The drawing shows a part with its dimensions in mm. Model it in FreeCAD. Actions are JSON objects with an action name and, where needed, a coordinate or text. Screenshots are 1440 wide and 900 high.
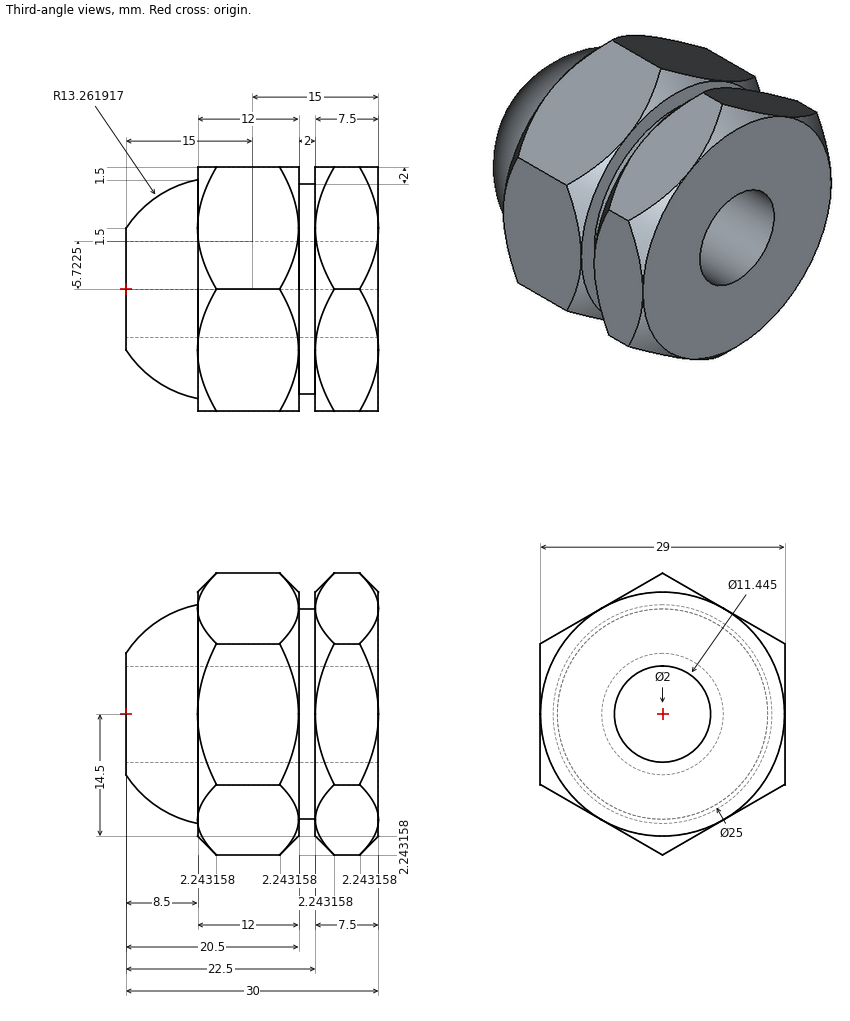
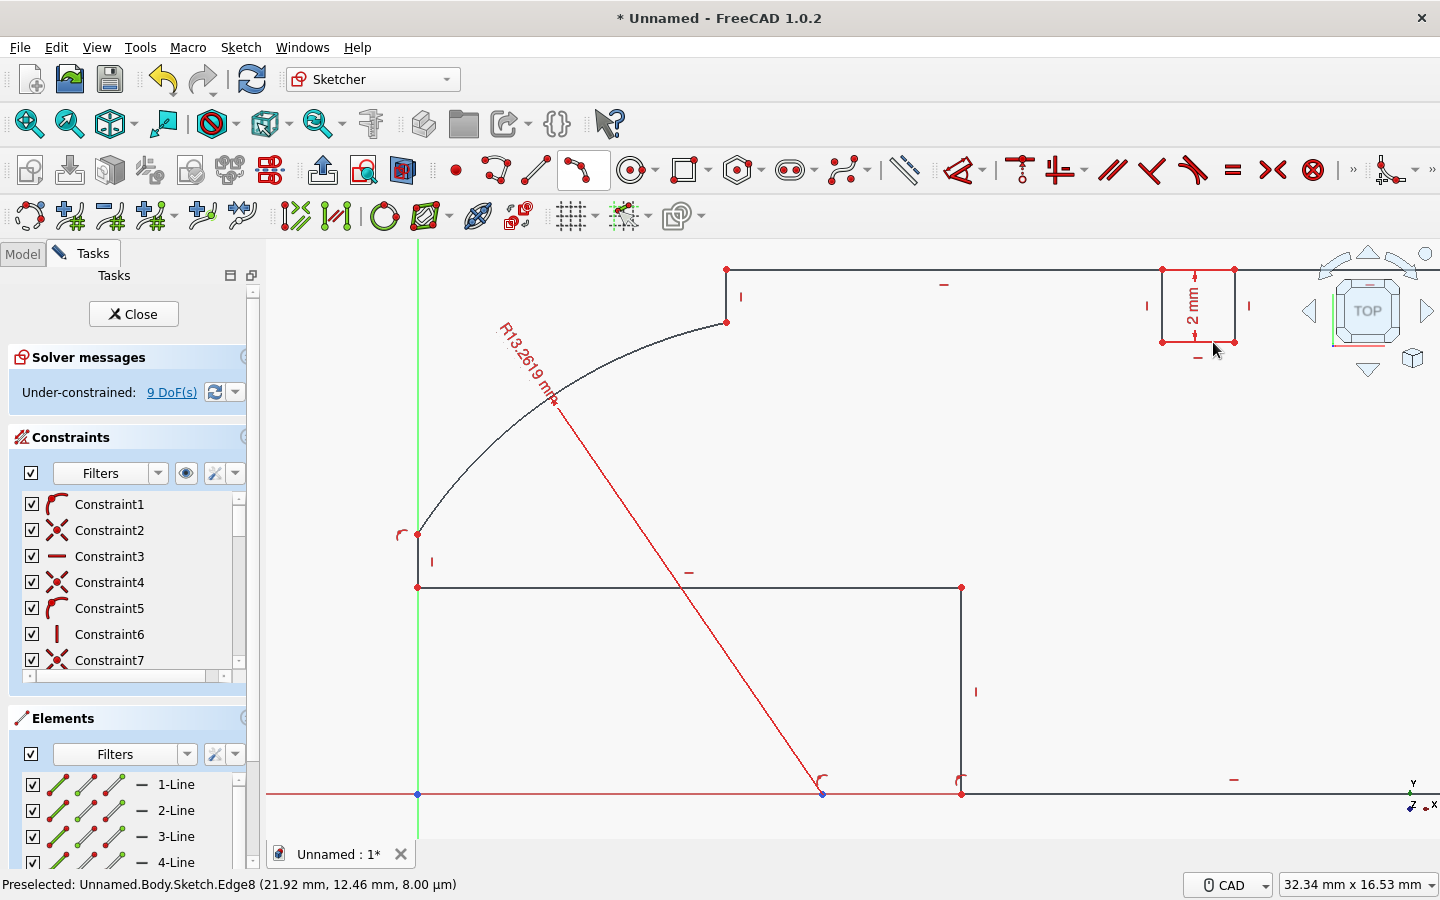
{"action": "key", "text": "l"}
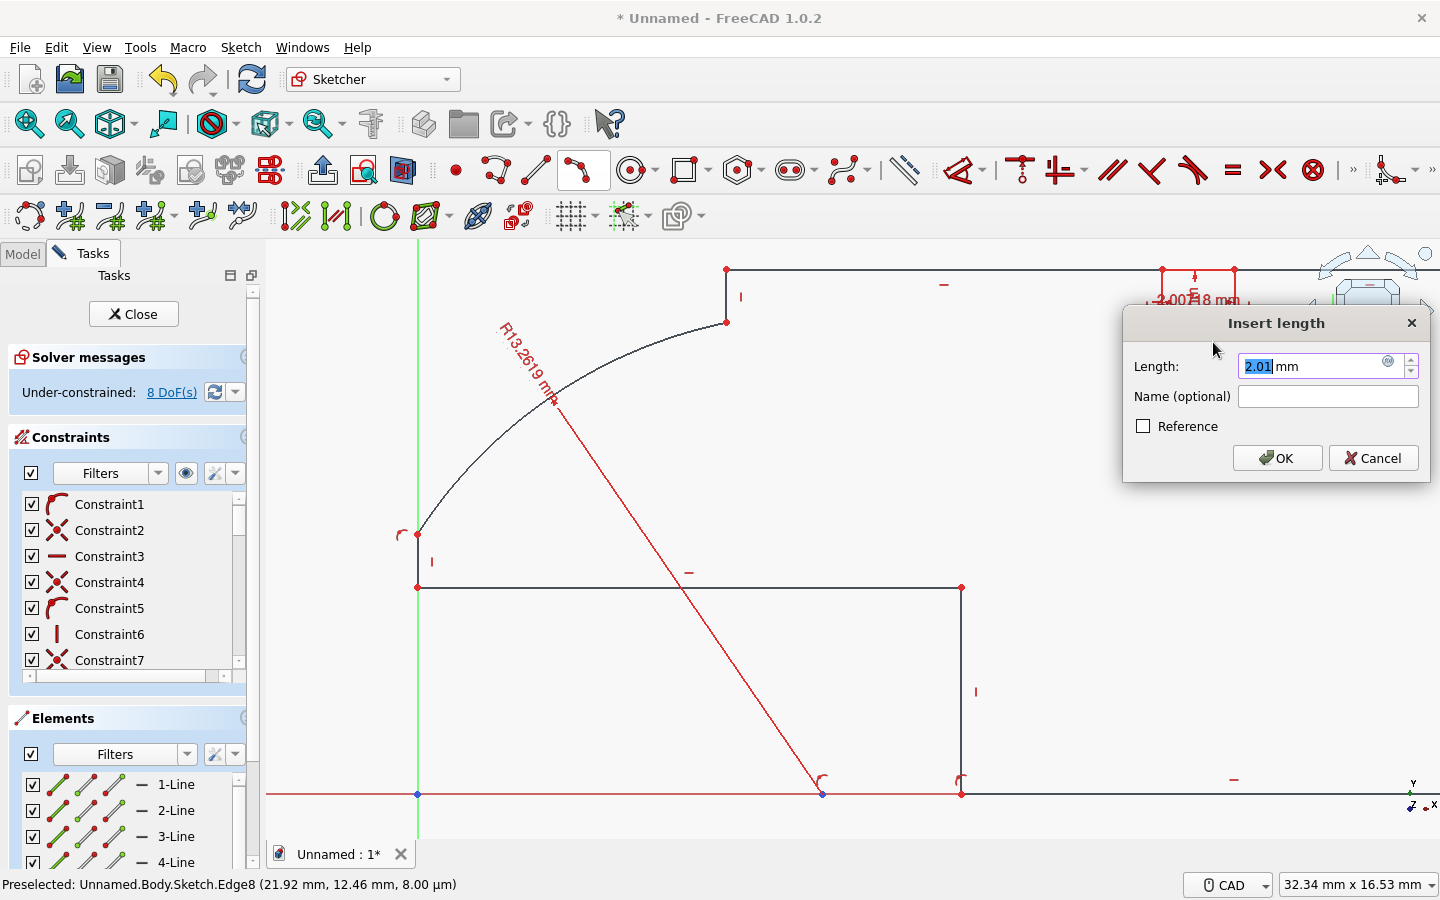
{"action": "type", "text": "2"}
{"action": "key", "text": "Return"}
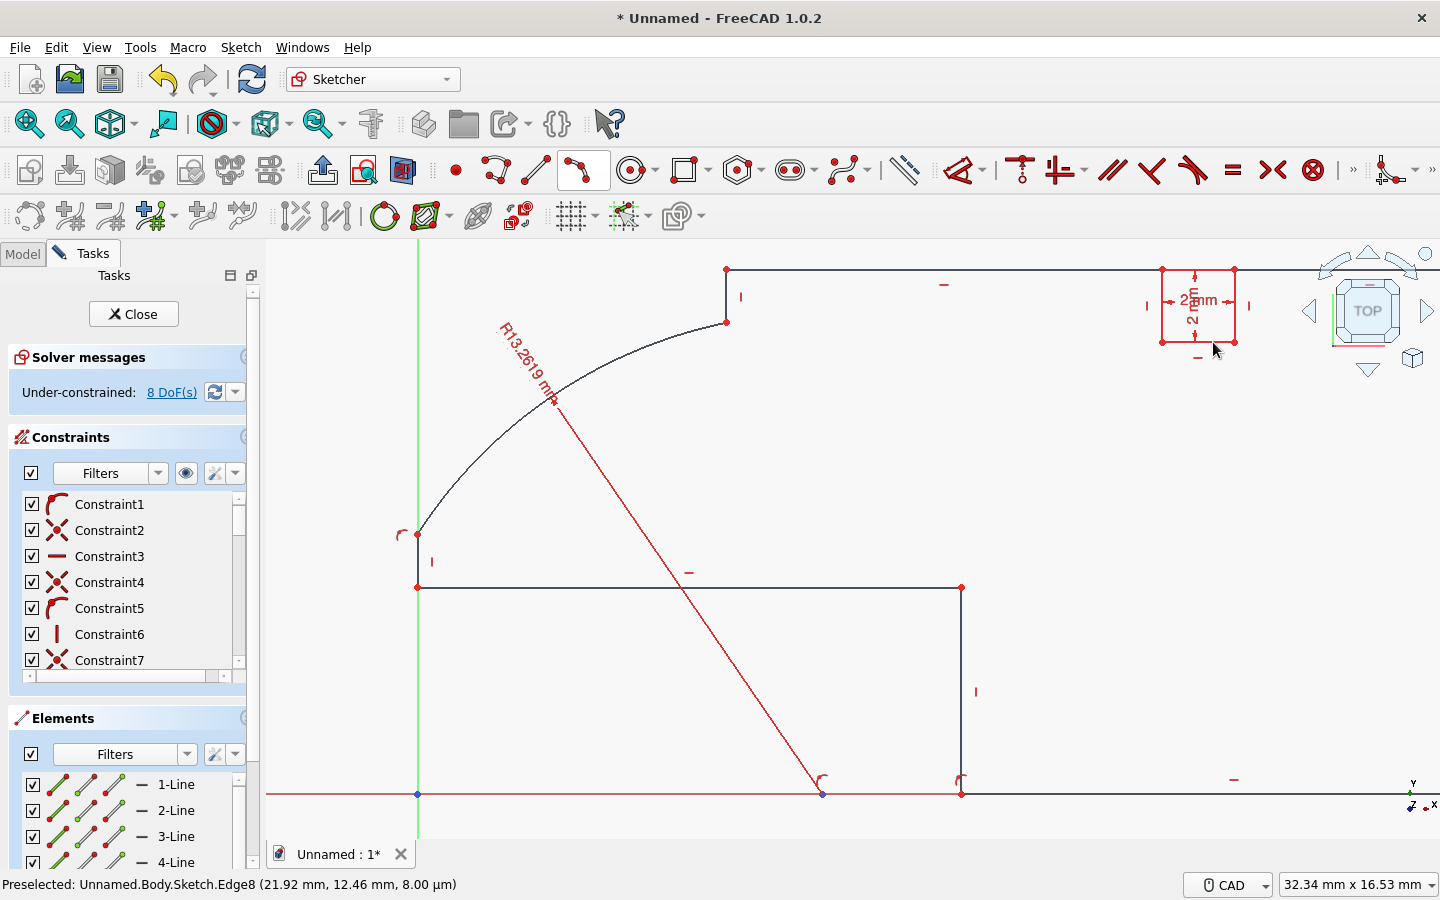
{"action": "left_click", "coordinate": [1162, 320]}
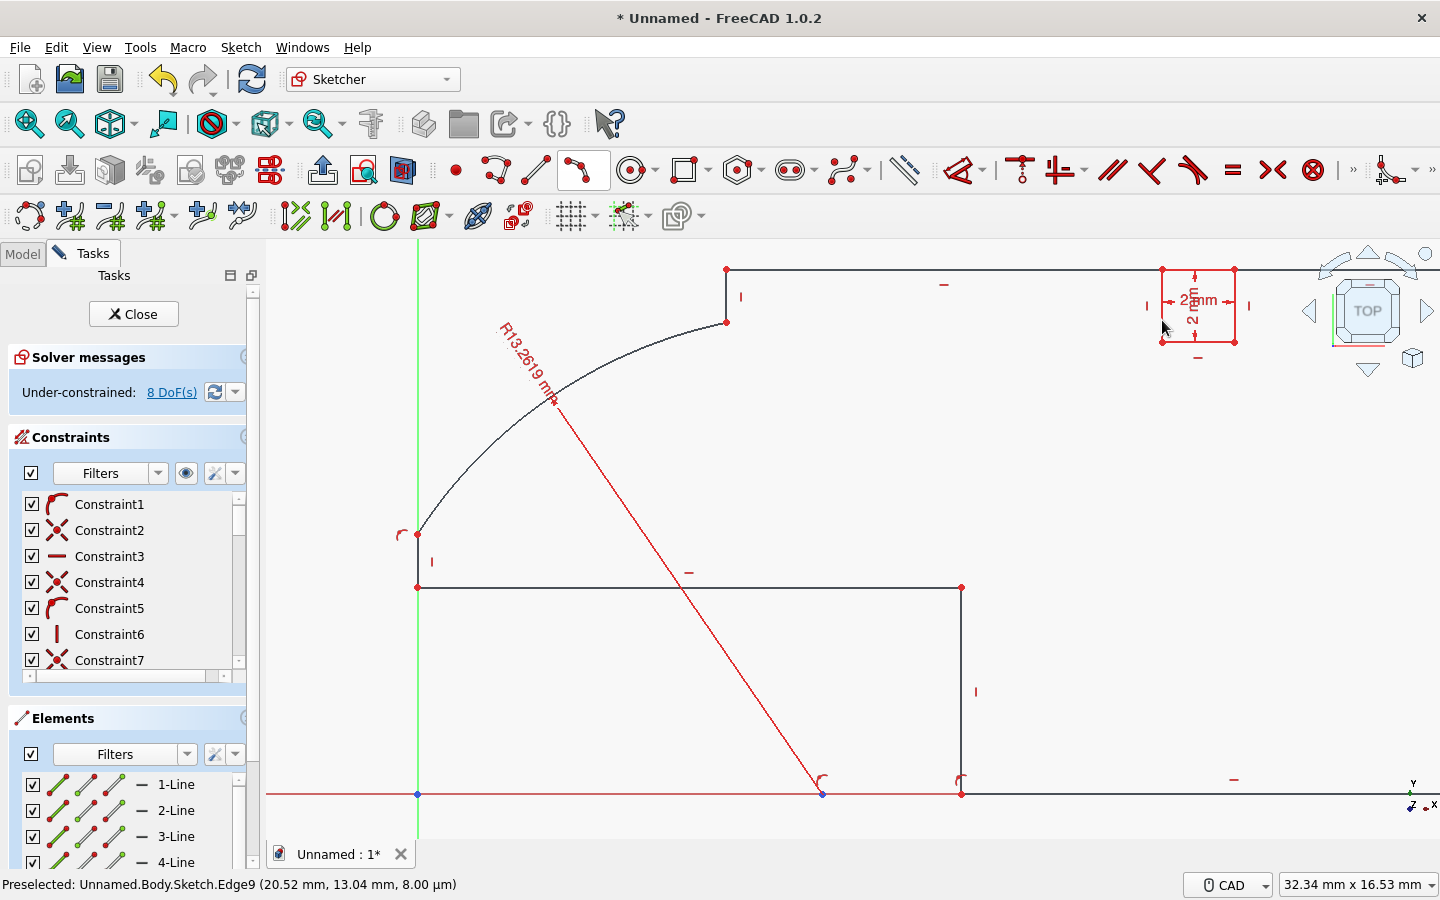
{"action": "left_click", "coordinate": [984, 170]}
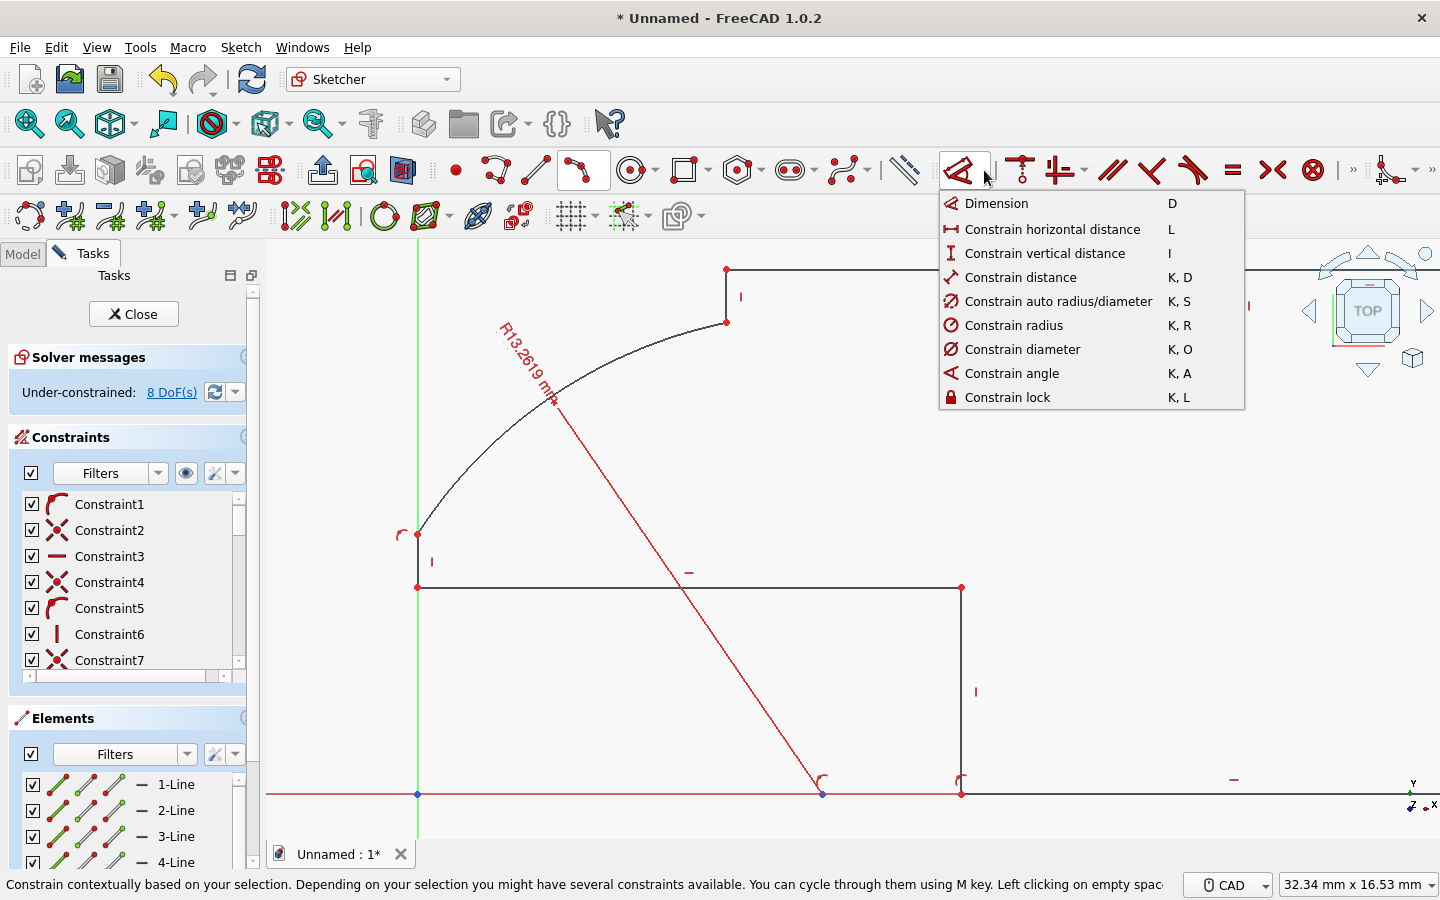
{"action": "left_click", "coordinate": [1092, 253]}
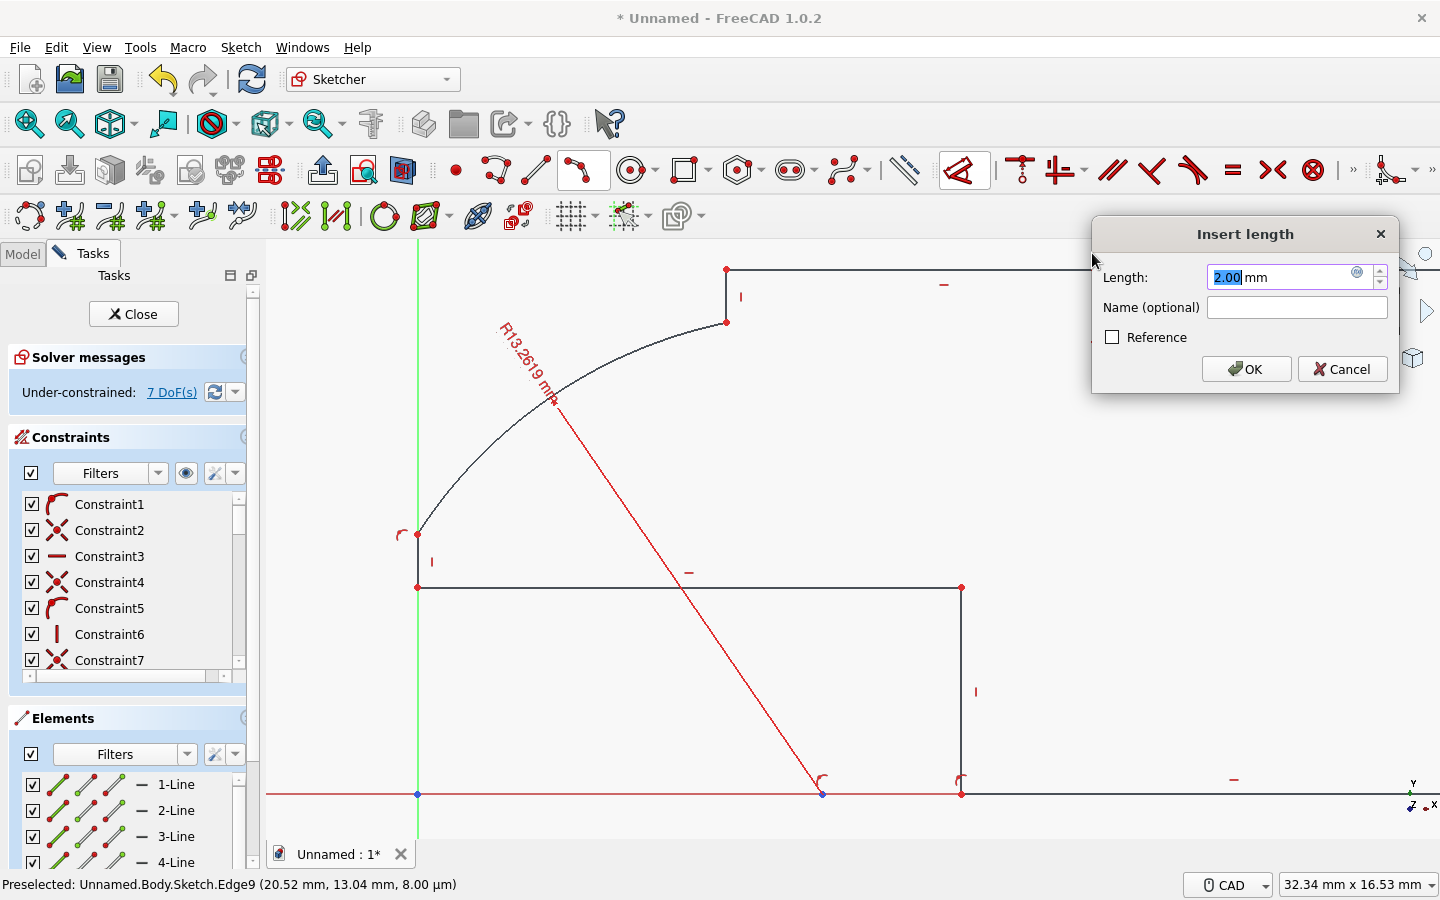
{"action": "type", "text": "2"}
{"action": "key", "text": "Return"}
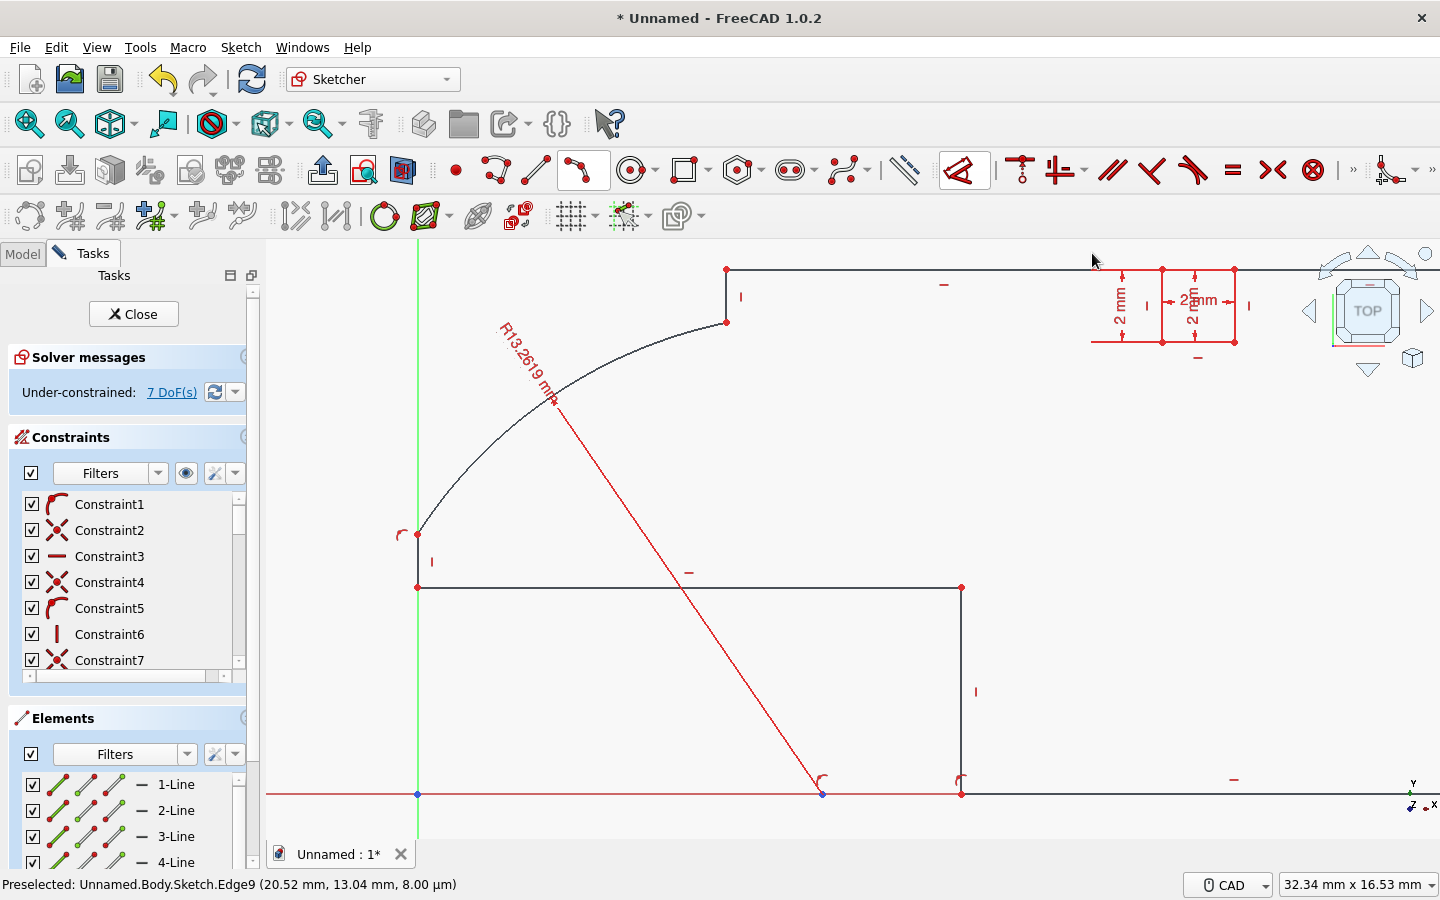
{"action": "left_click", "coordinate": [581, 588]}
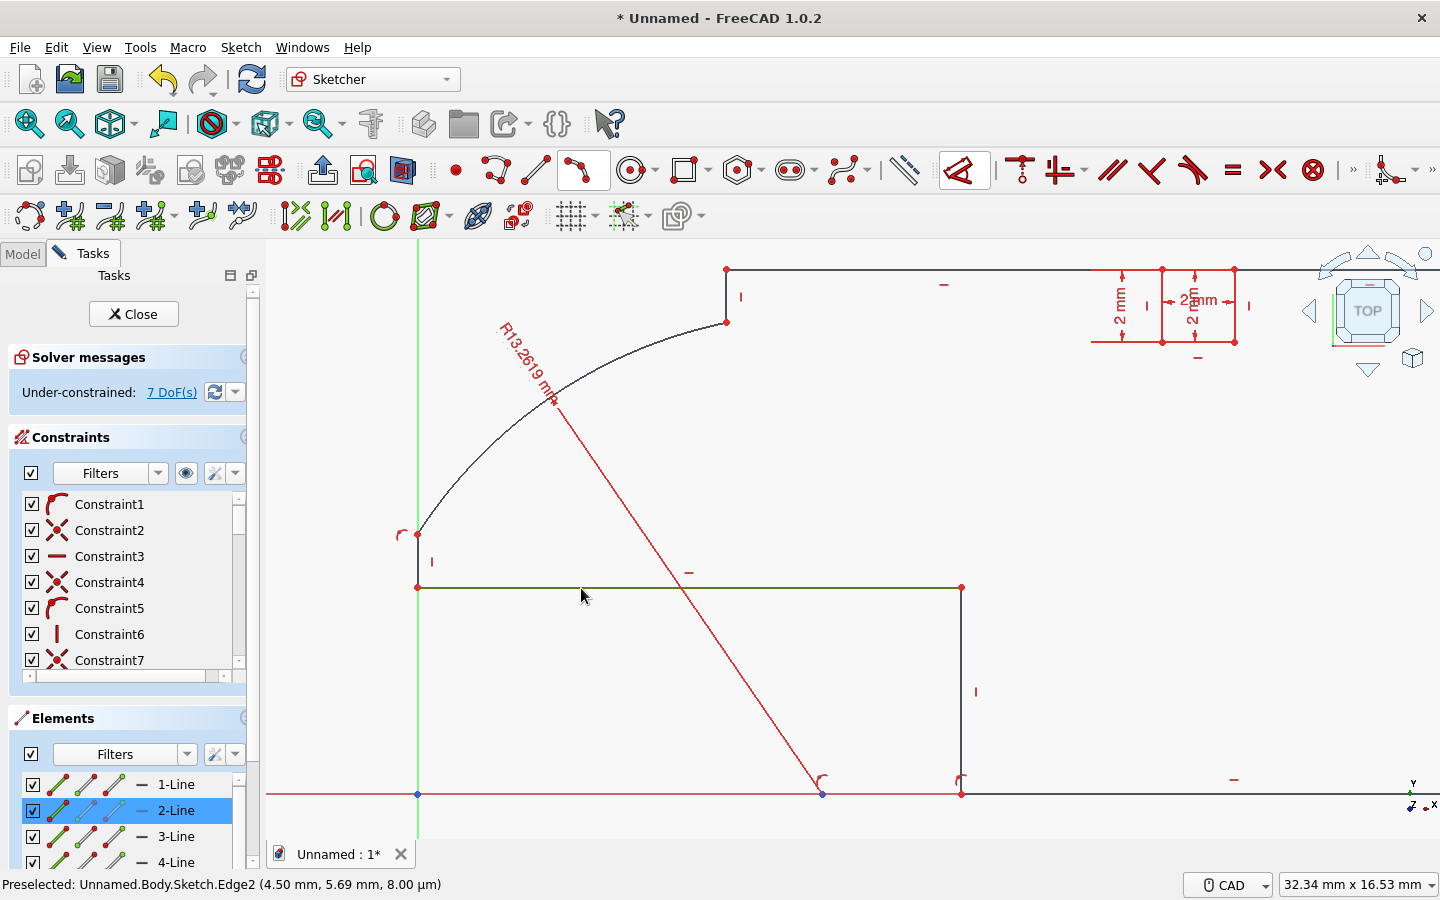
{"action": "left_click", "coordinate": [984, 170]}